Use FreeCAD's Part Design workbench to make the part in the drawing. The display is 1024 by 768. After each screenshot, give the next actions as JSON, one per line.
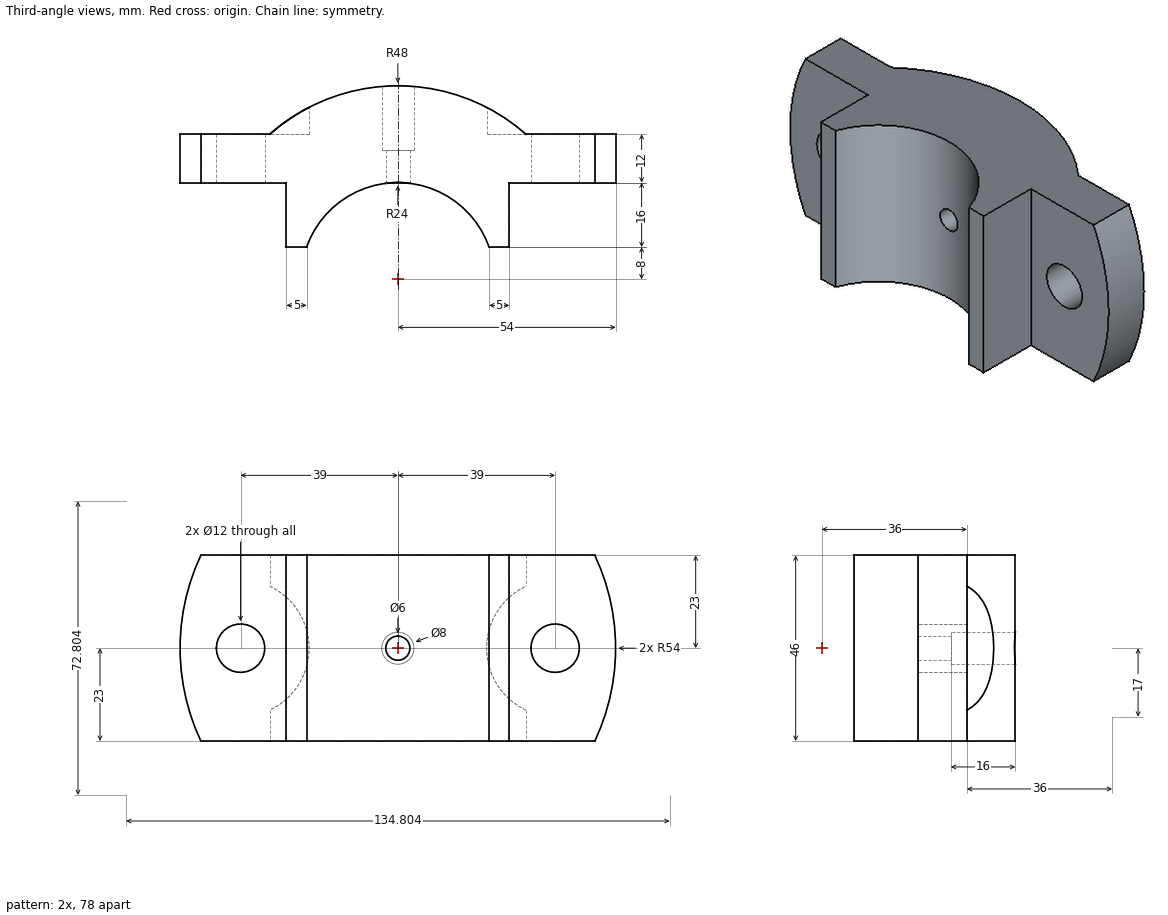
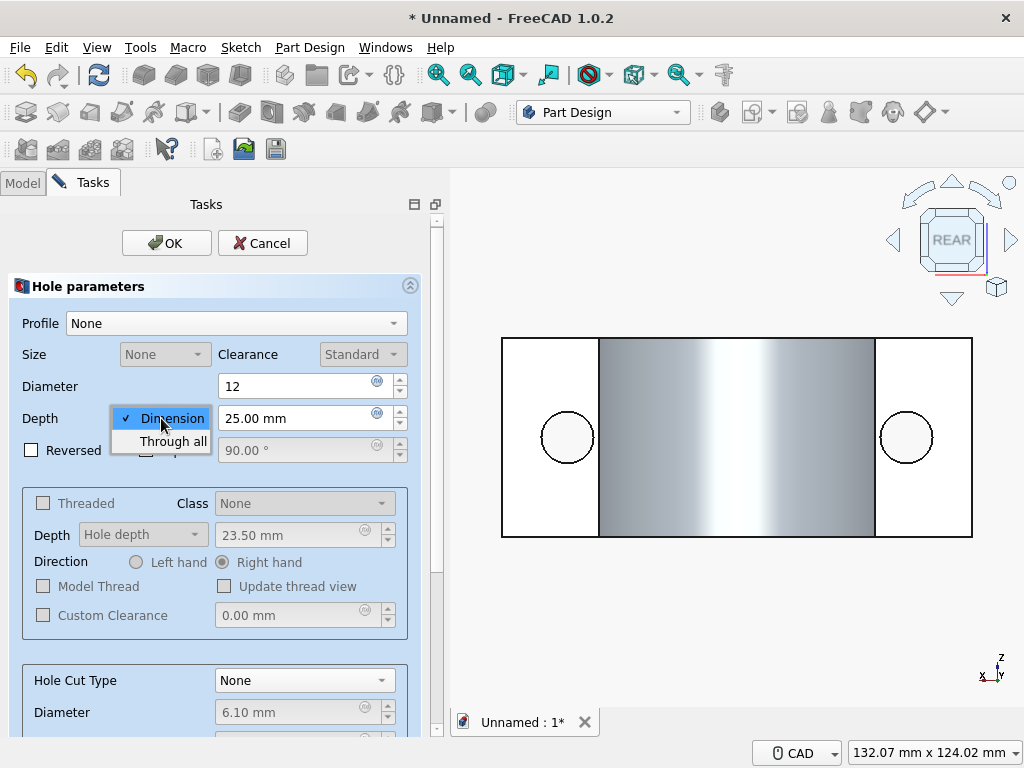
{"action": "left_click", "coordinate": [160, 442]}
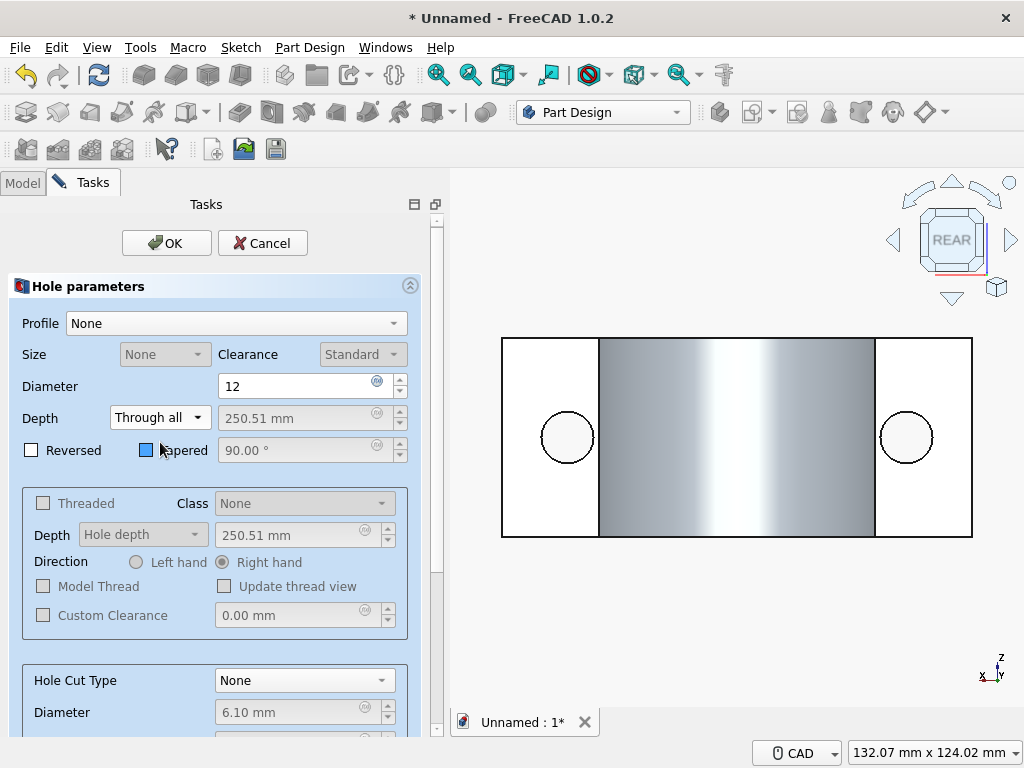
{"action": "left_click", "coordinate": [167, 243]}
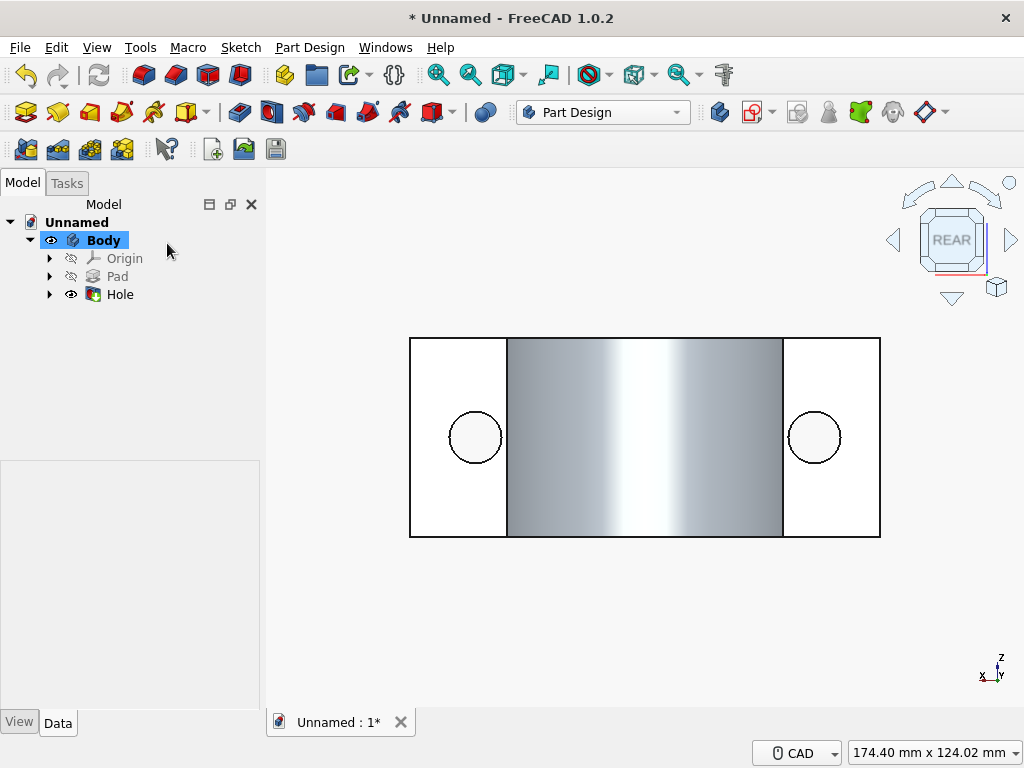
{"action": "left_click", "coordinate": [50, 258]}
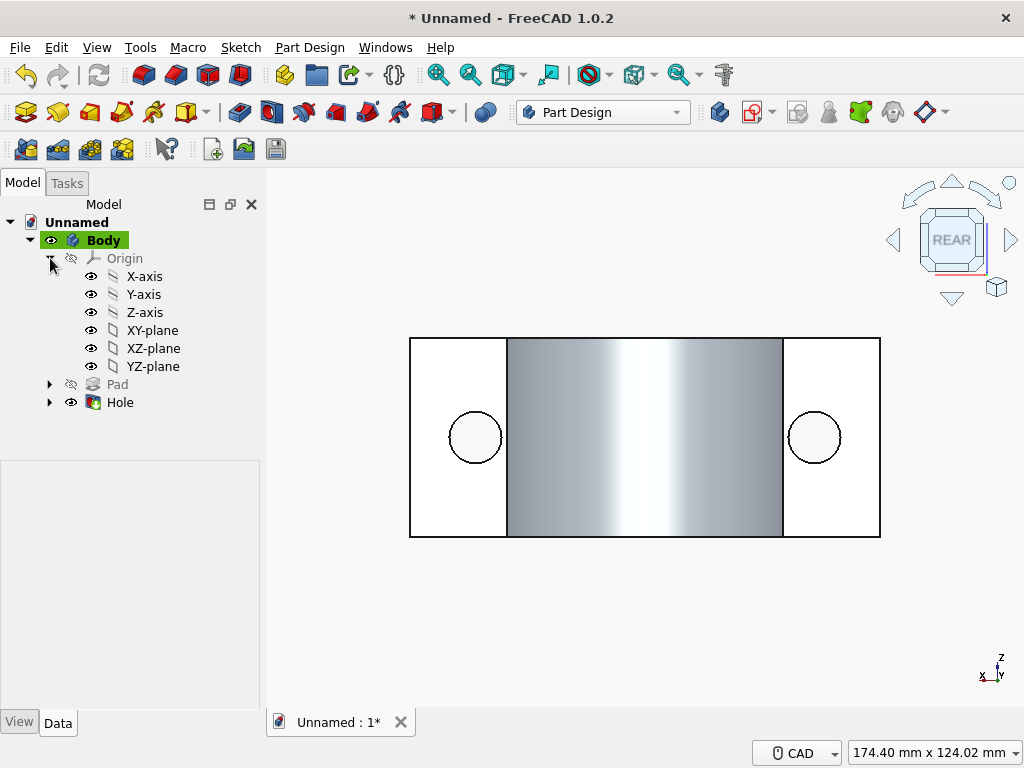
{"action": "left_click", "coordinate": [136, 366]}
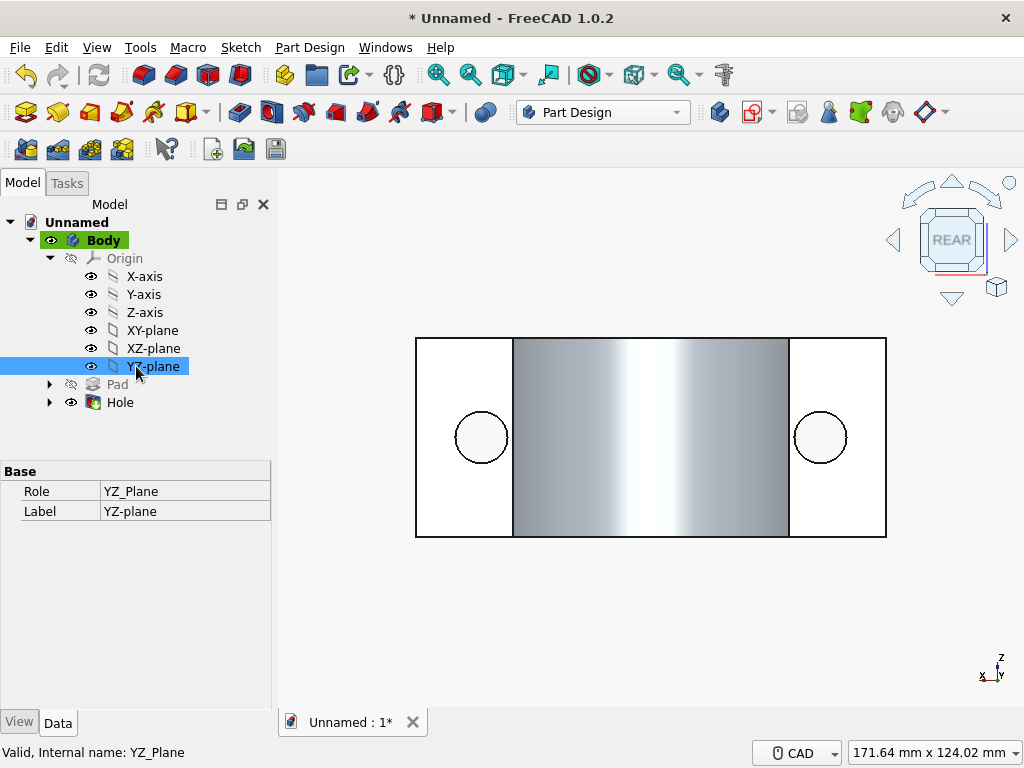
{"action": "left_click", "coordinate": [926, 112]}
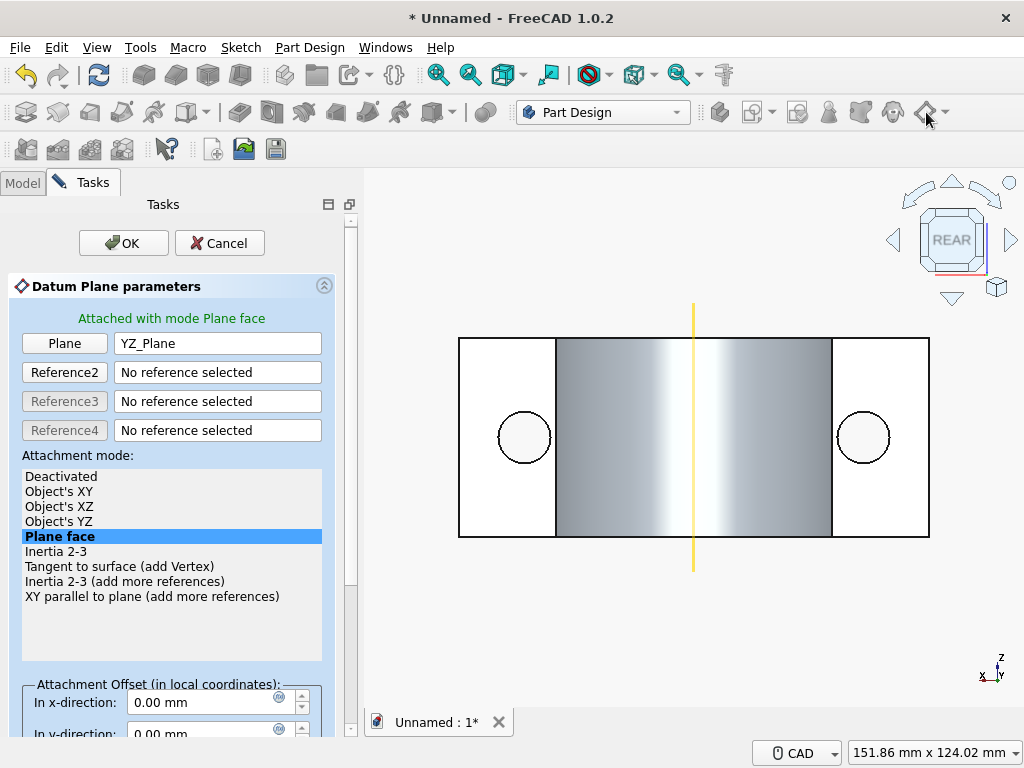
{"action": "scroll", "coordinate": [351, 475], "scroll_direction": "down", "scroll_amount": 2}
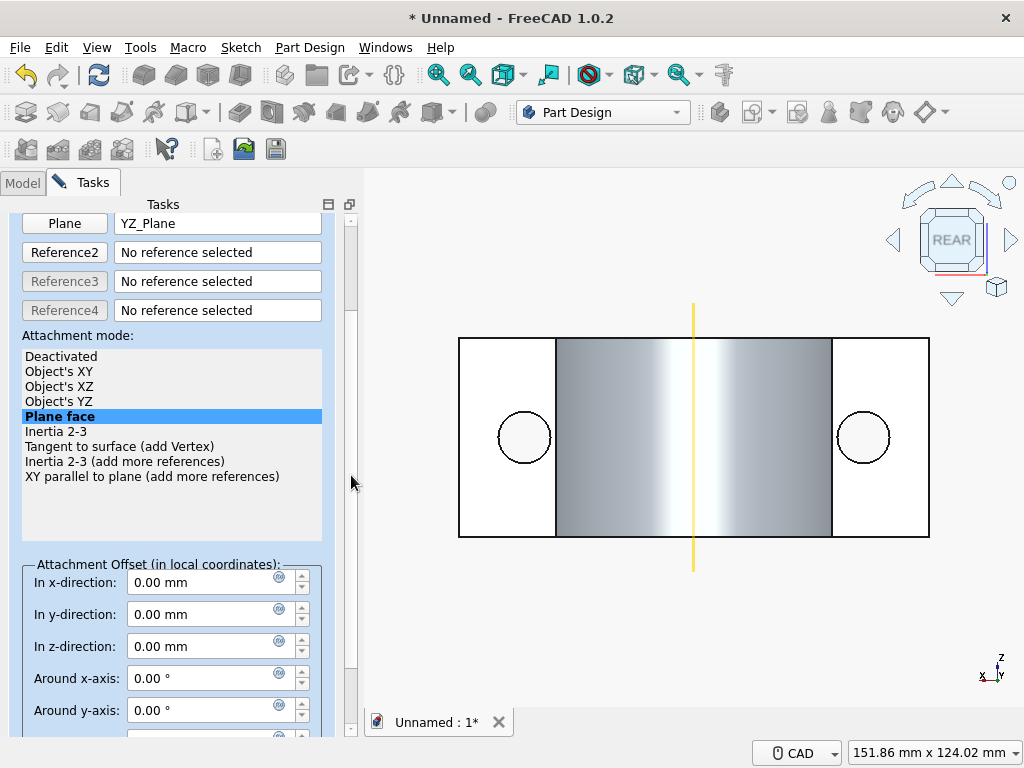
{"action": "triple_click", "coordinate": [210, 646]}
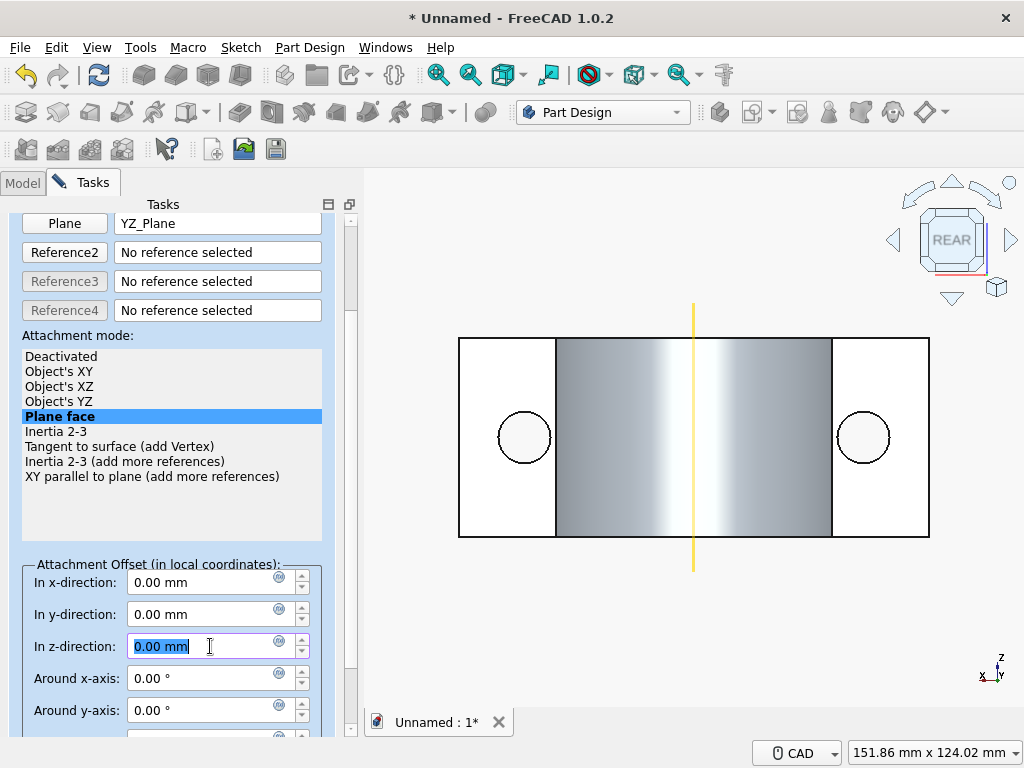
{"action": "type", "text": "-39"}
{"action": "key", "text": "Tab"}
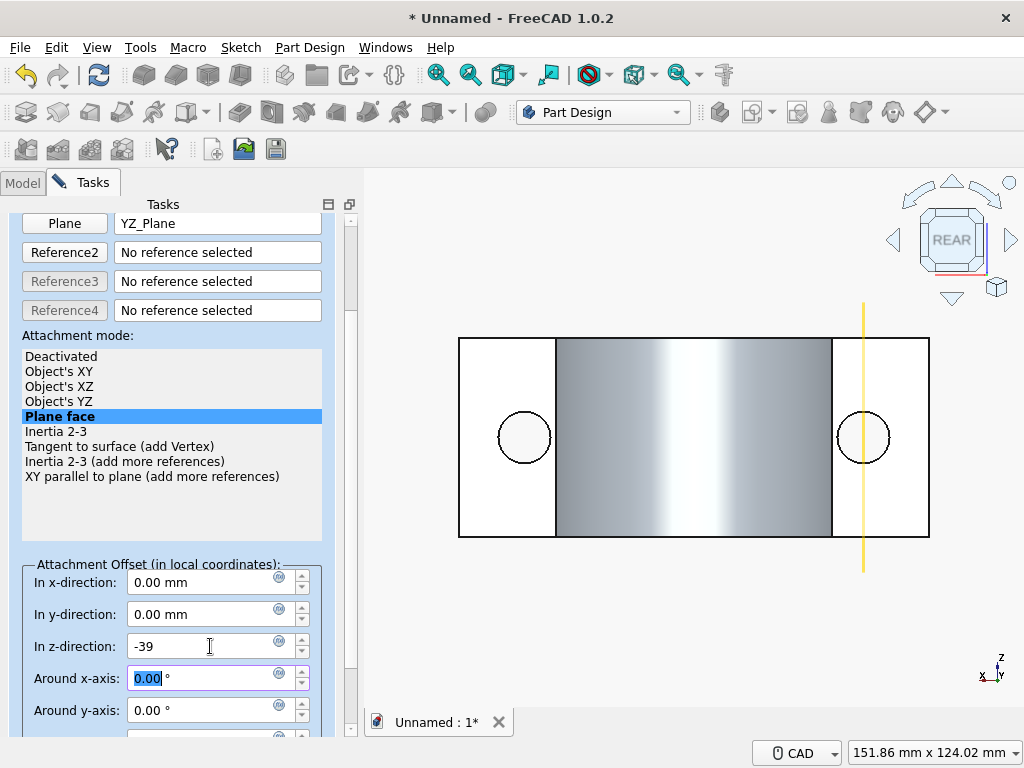
{"action": "scroll", "coordinate": [351, 475], "scroll_direction": "up", "scroll_amount": 3}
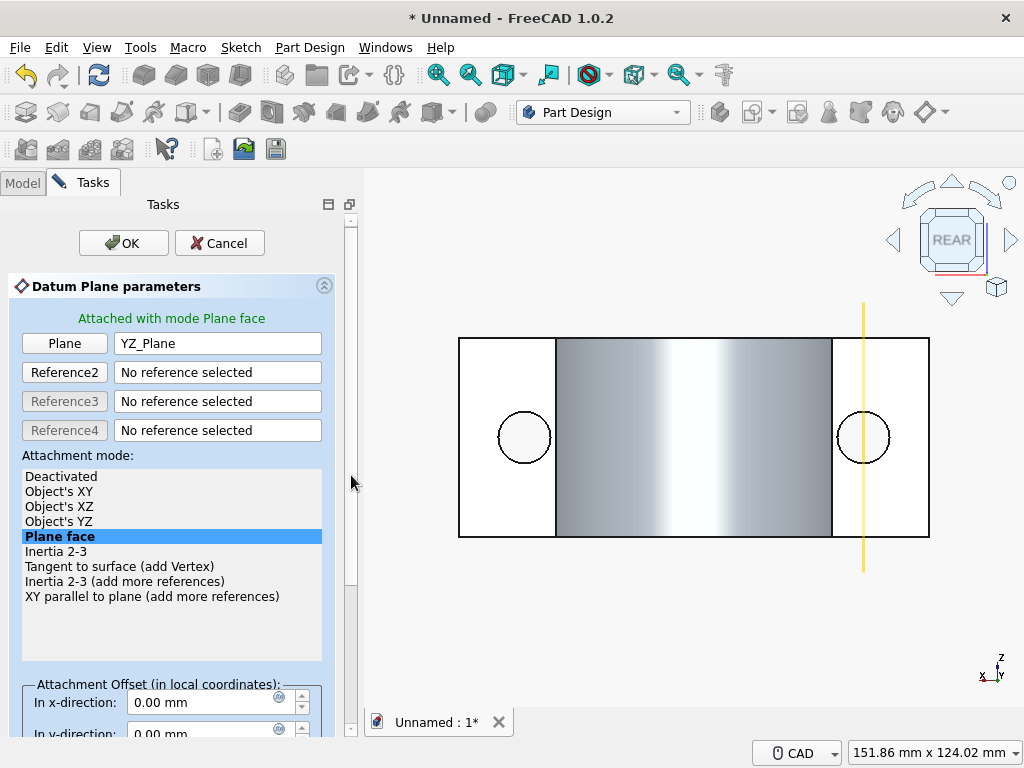
{"action": "left_click", "coordinate": [124, 243]}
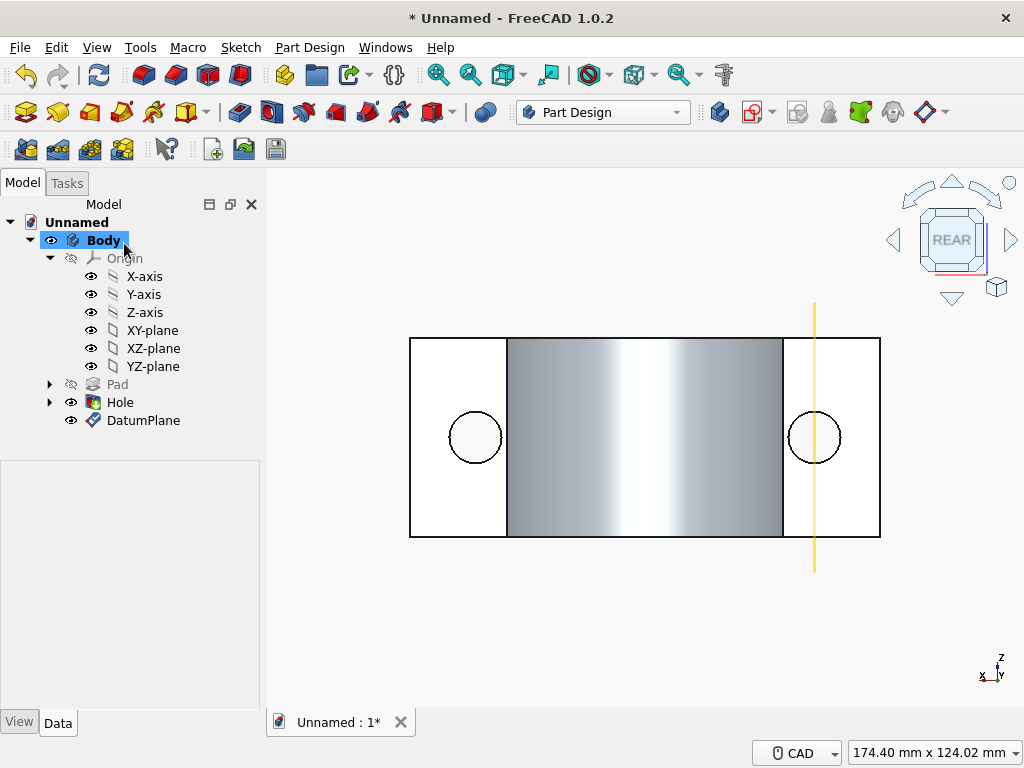
{"action": "left_click", "coordinate": [116, 420]}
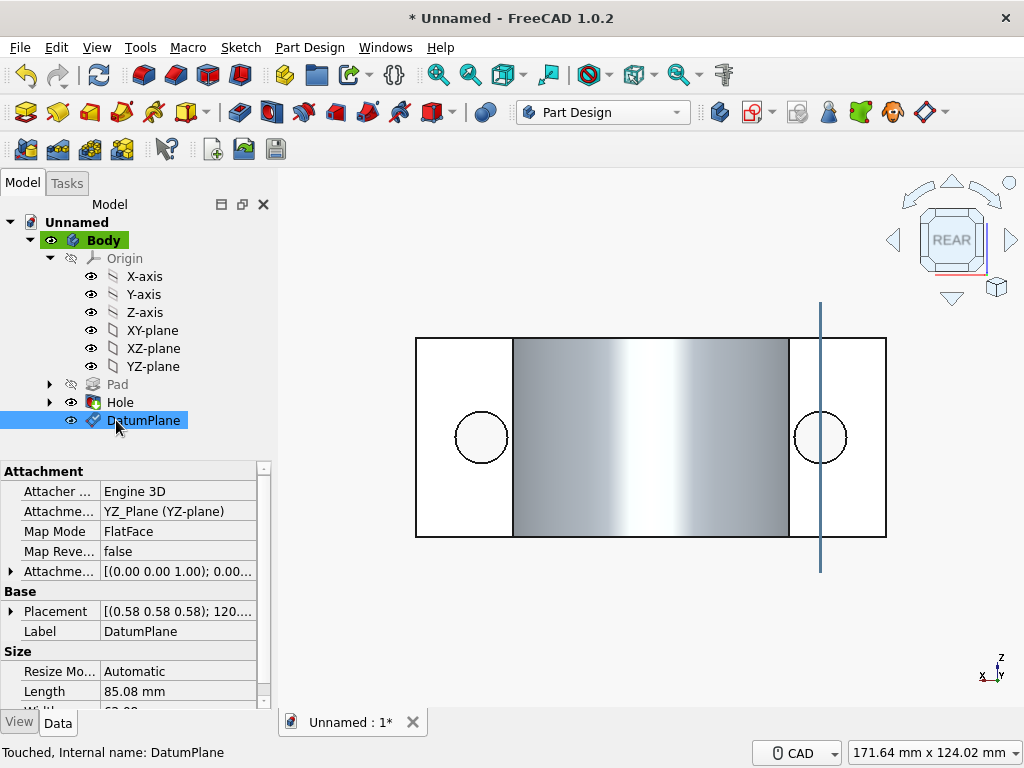
{"action": "left_click", "coordinate": [752, 112]}